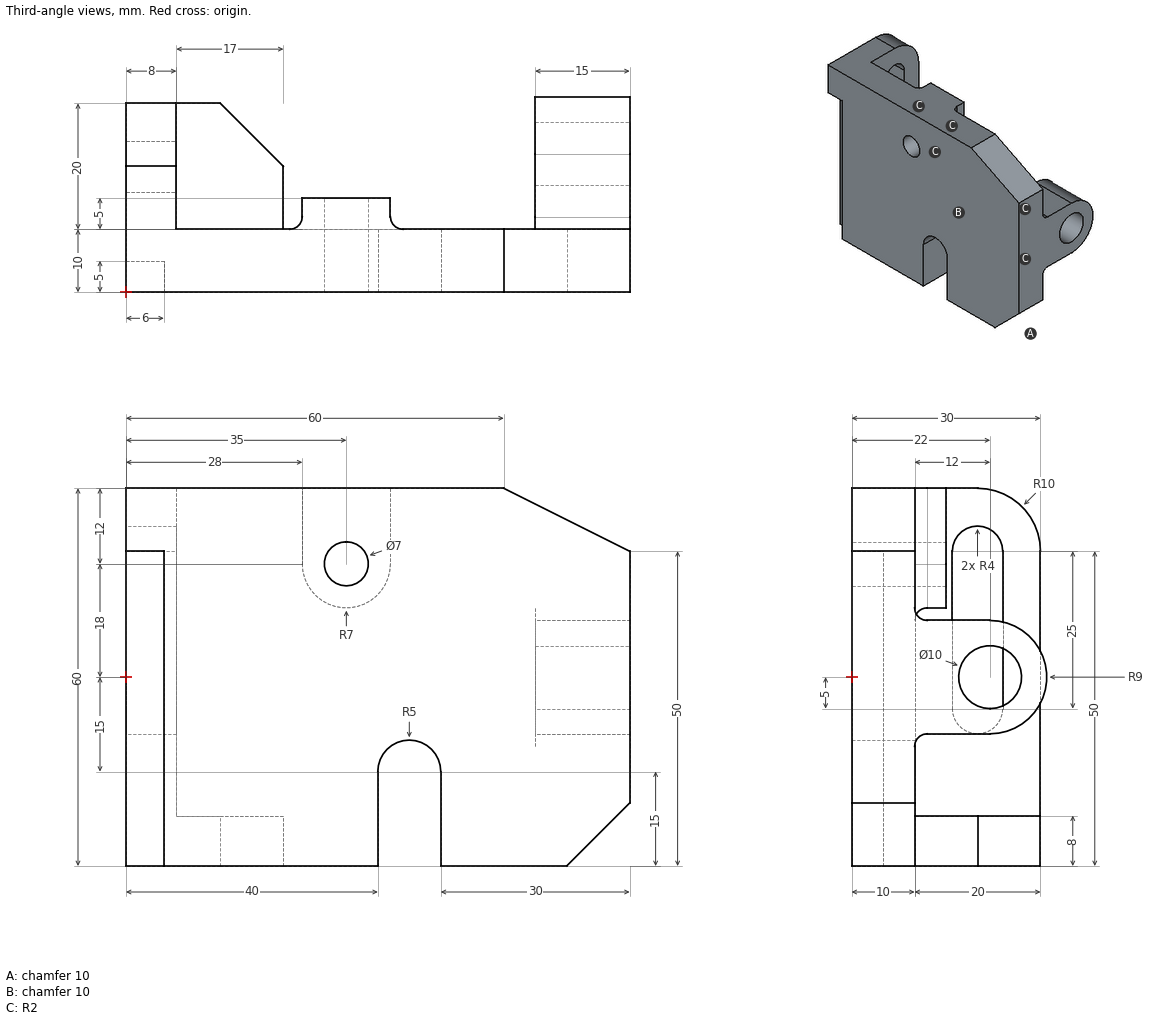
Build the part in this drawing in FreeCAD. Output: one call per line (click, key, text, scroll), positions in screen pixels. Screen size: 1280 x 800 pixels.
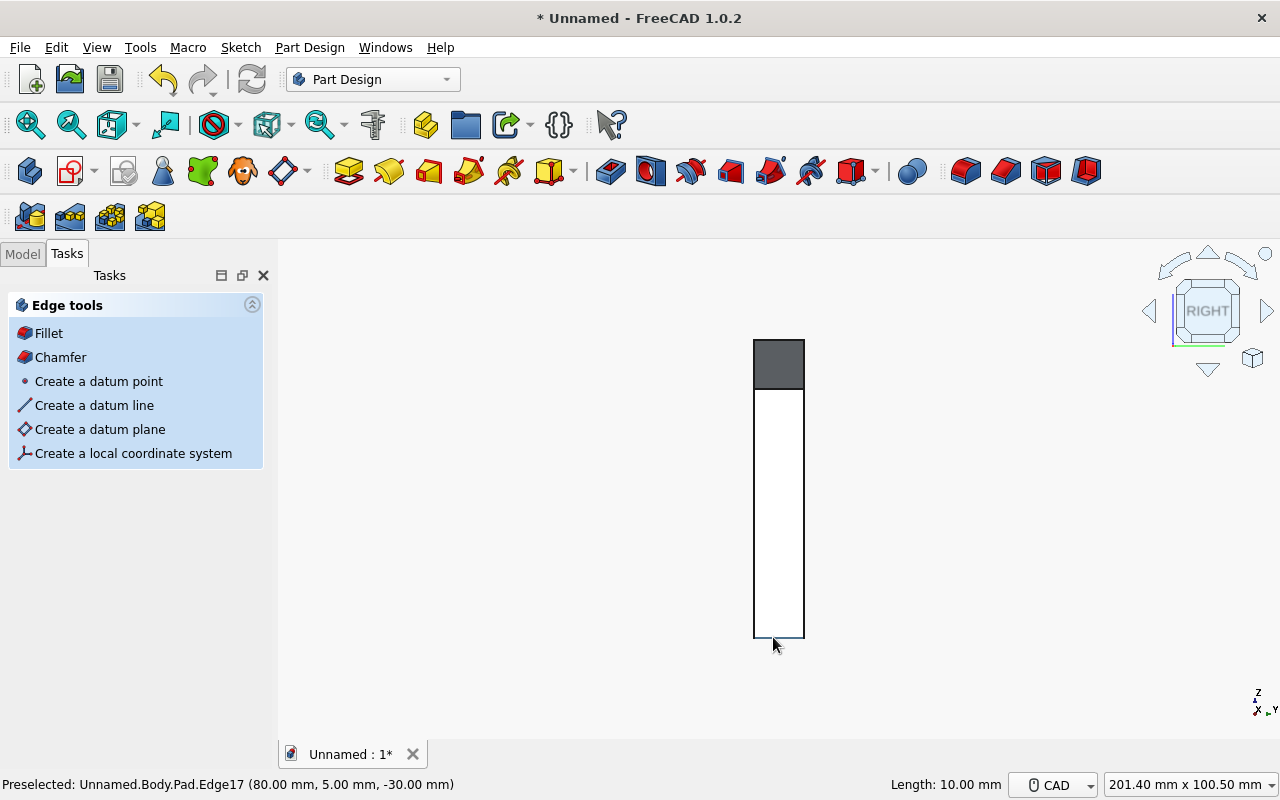
click(1006, 172)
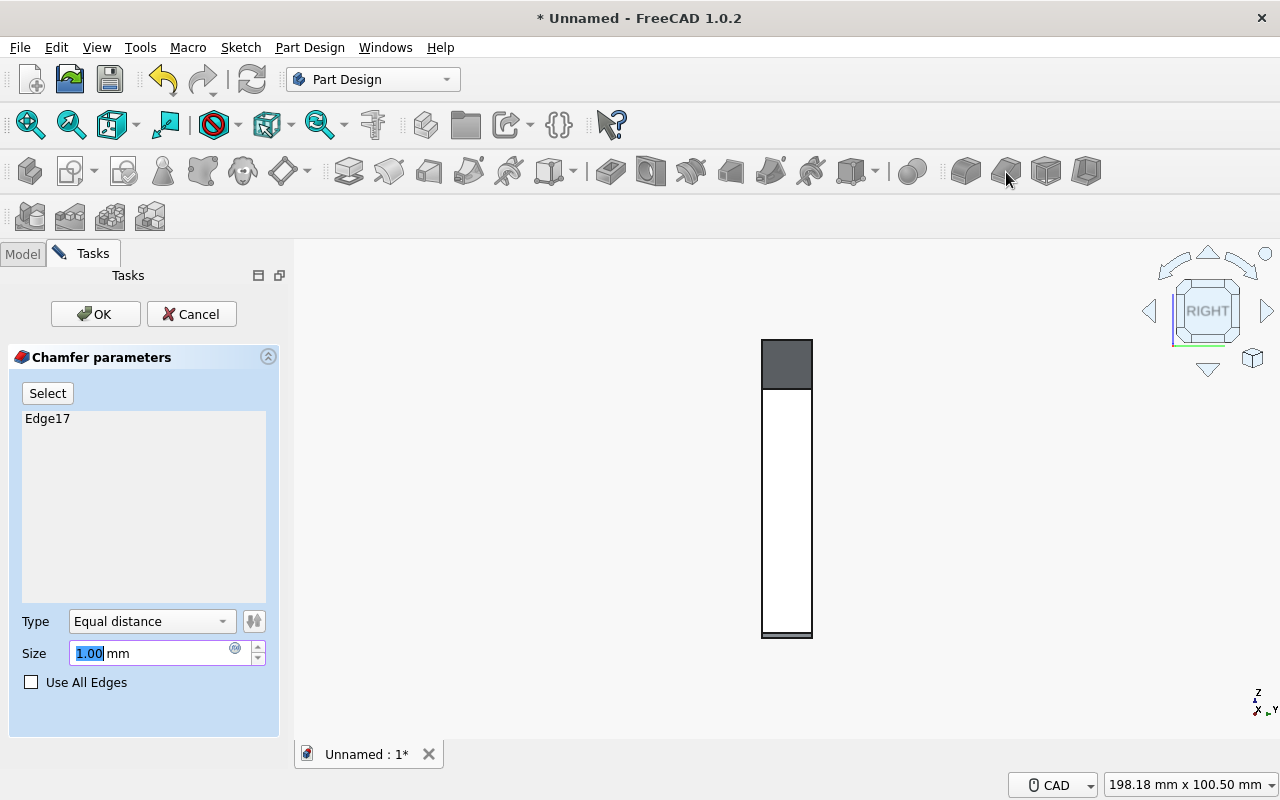
text(10)
key(Tab)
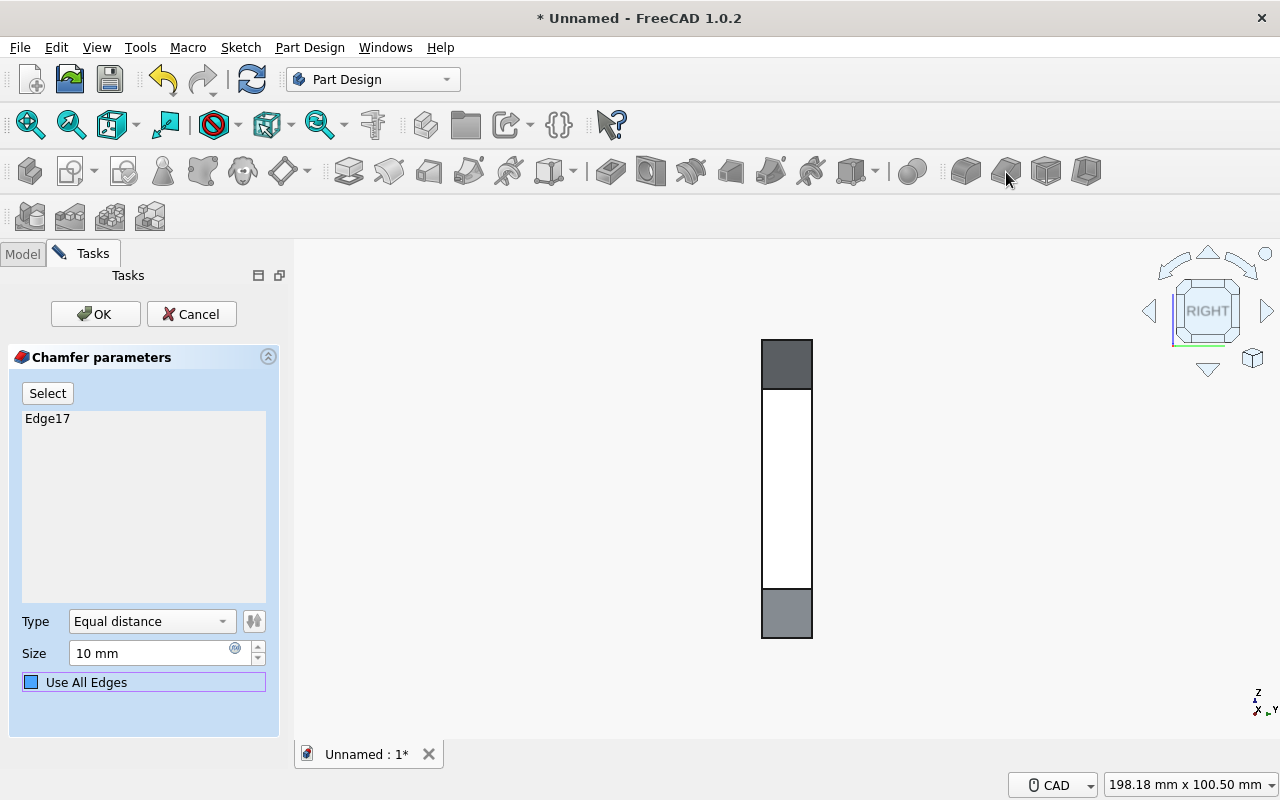
click(96, 314)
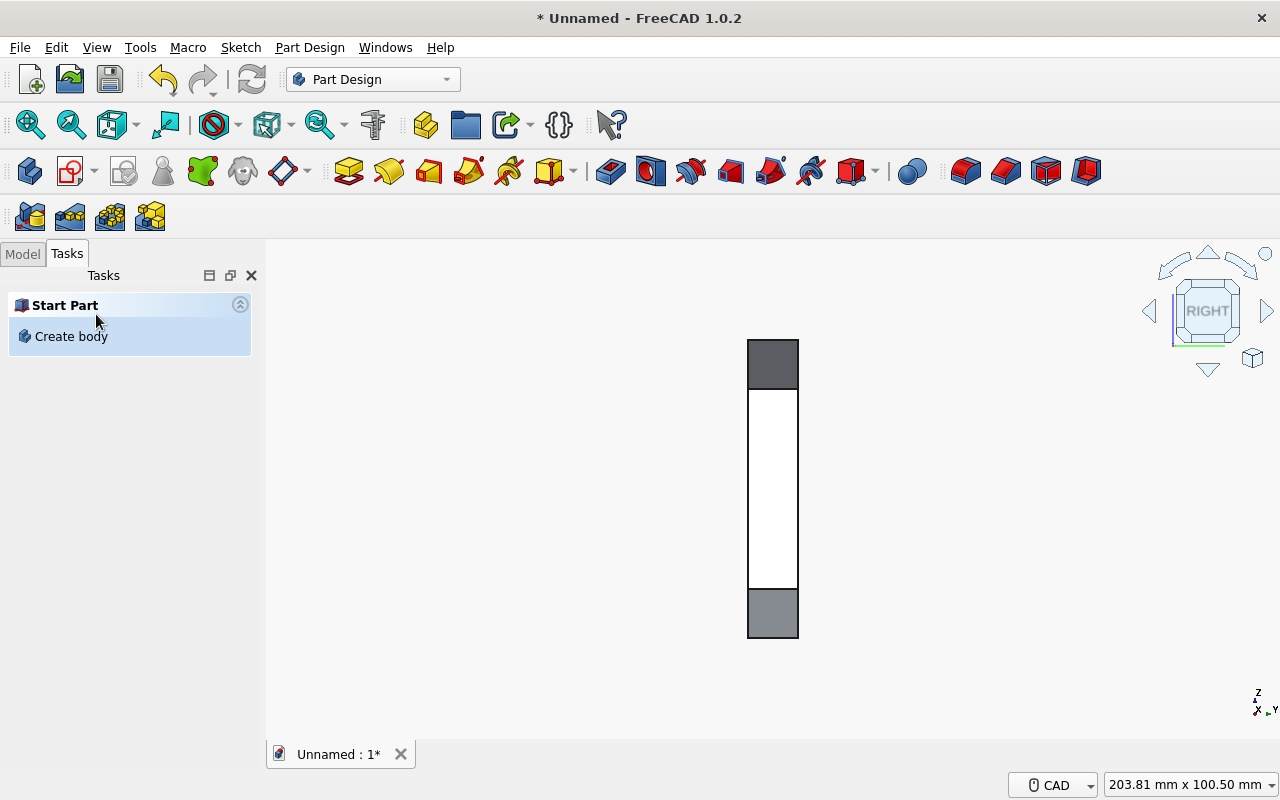
click(70, 172)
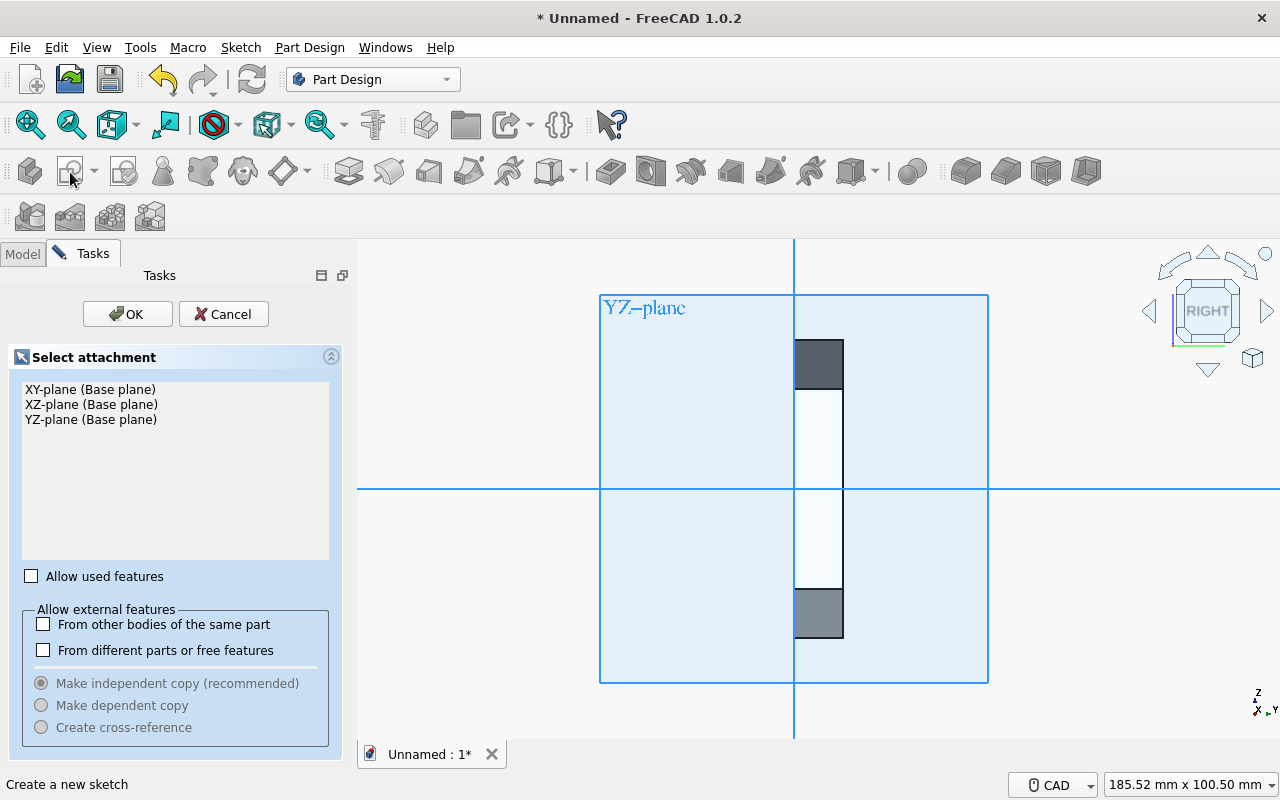
click(82, 420)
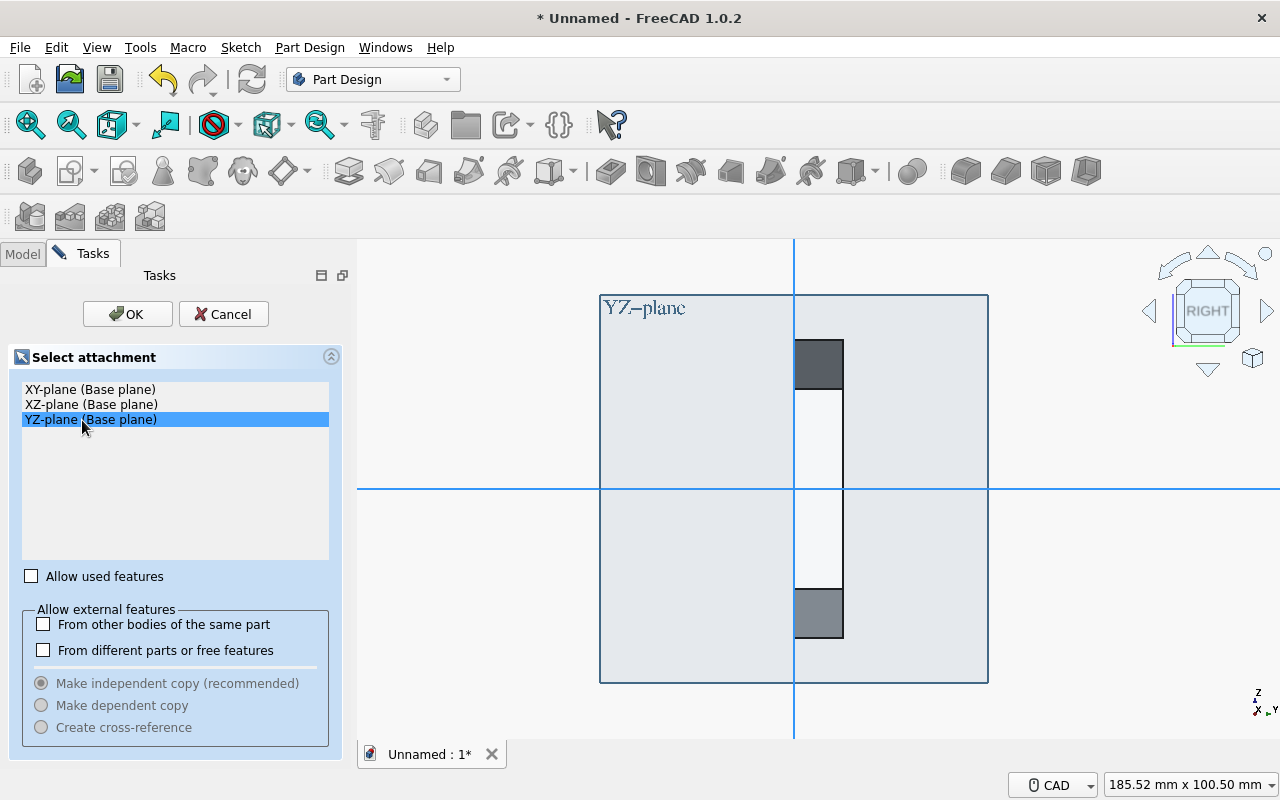
click(128, 314)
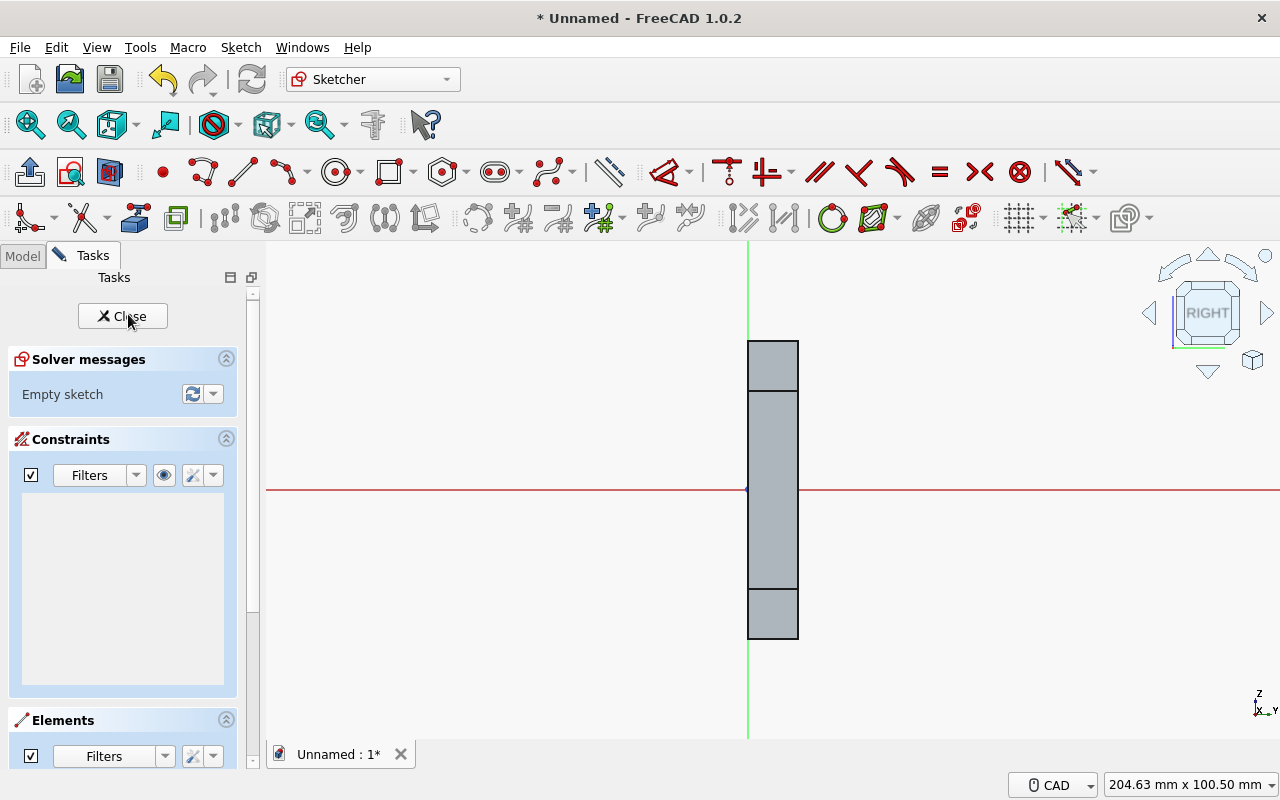
click(110, 172)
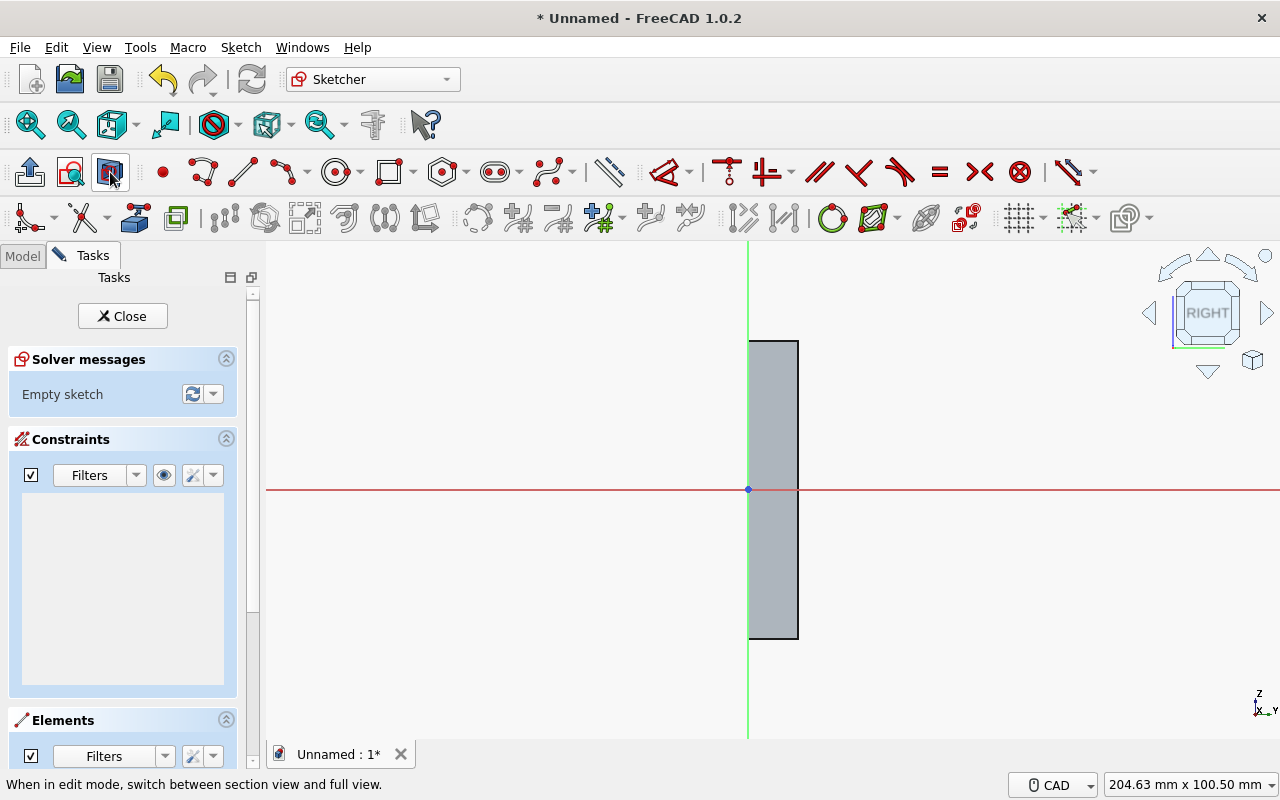
click(204, 172)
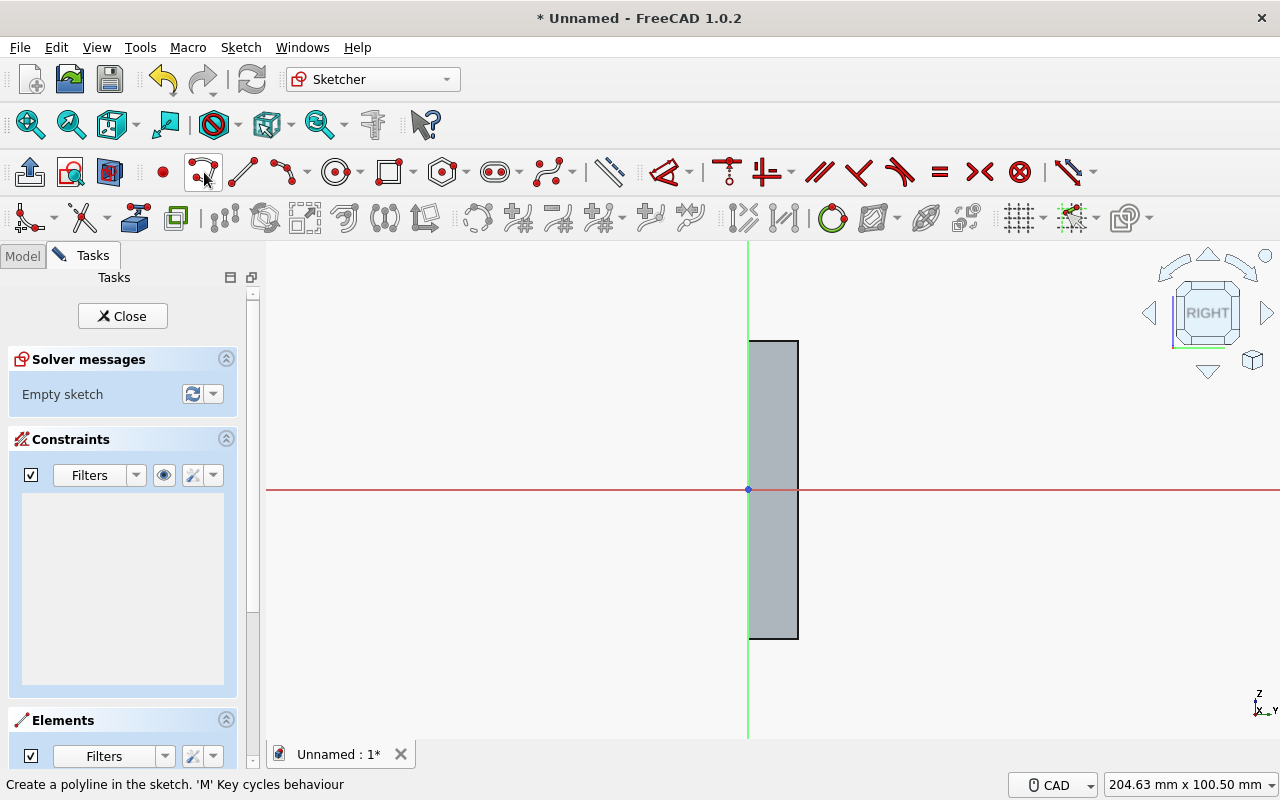
click(897, 391)
click(897, 639)
click(798, 639)
click(798, 341)
click(847, 341)
right_click(847, 341)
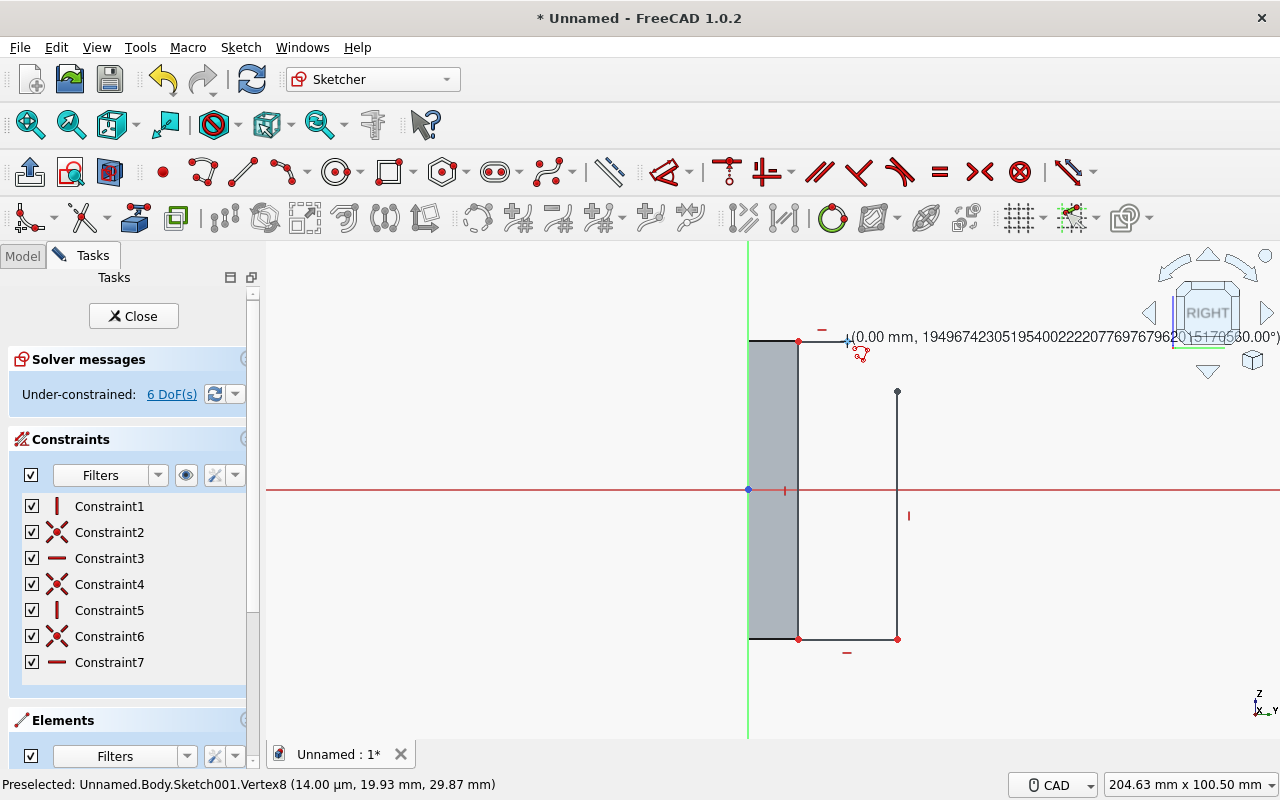
key(g)
key(3)
key(a)